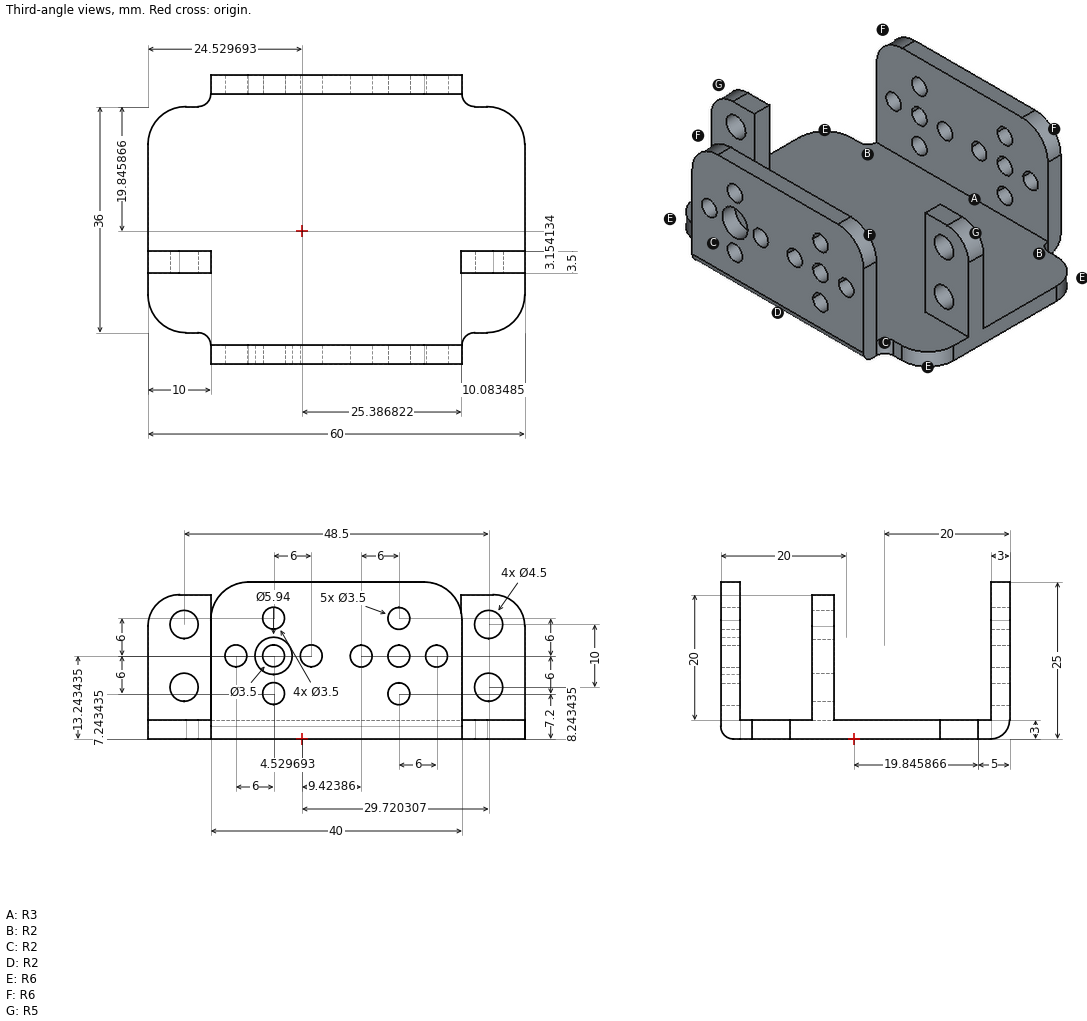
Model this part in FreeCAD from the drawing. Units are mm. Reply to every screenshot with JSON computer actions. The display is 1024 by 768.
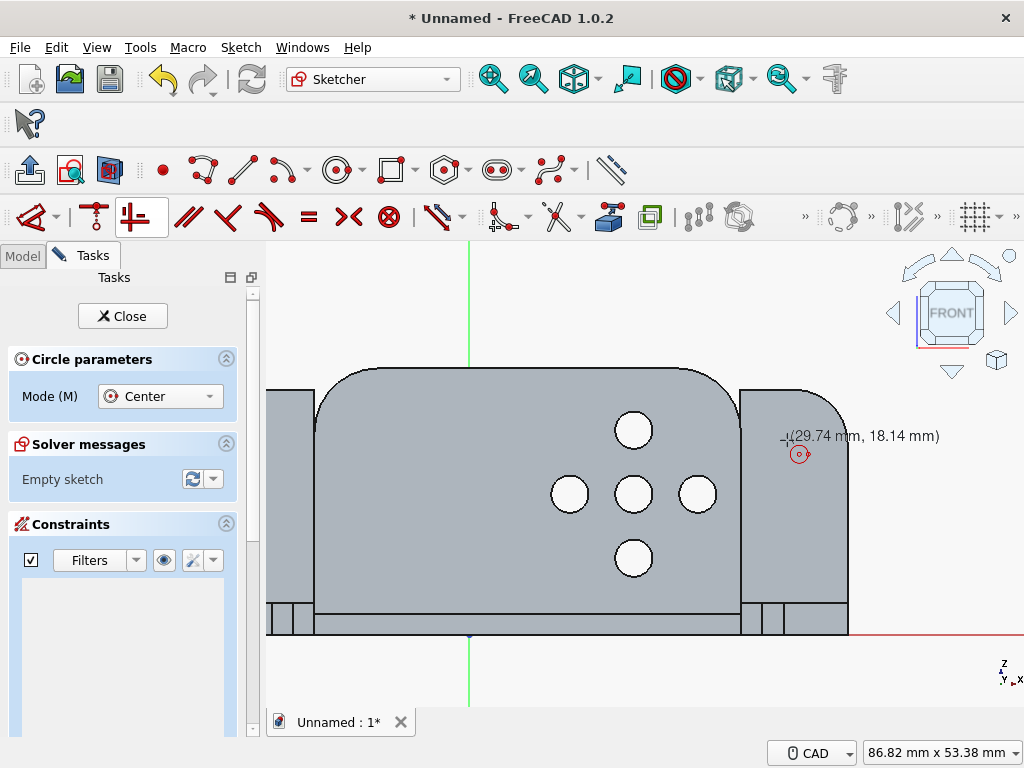
{"action": "left_click", "coordinate": [786, 440]}
{"action": "left_click", "coordinate": [803, 423]}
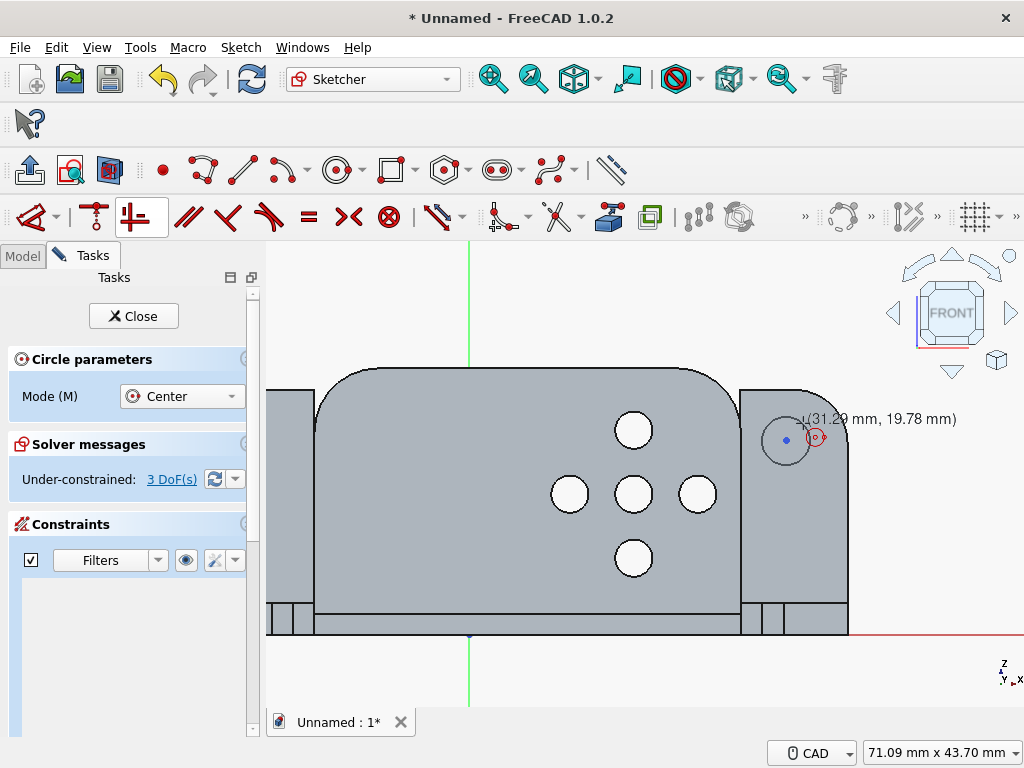
{"action": "left_click", "coordinate": [786, 547]}
{"action": "left_click", "coordinate": [803, 530]}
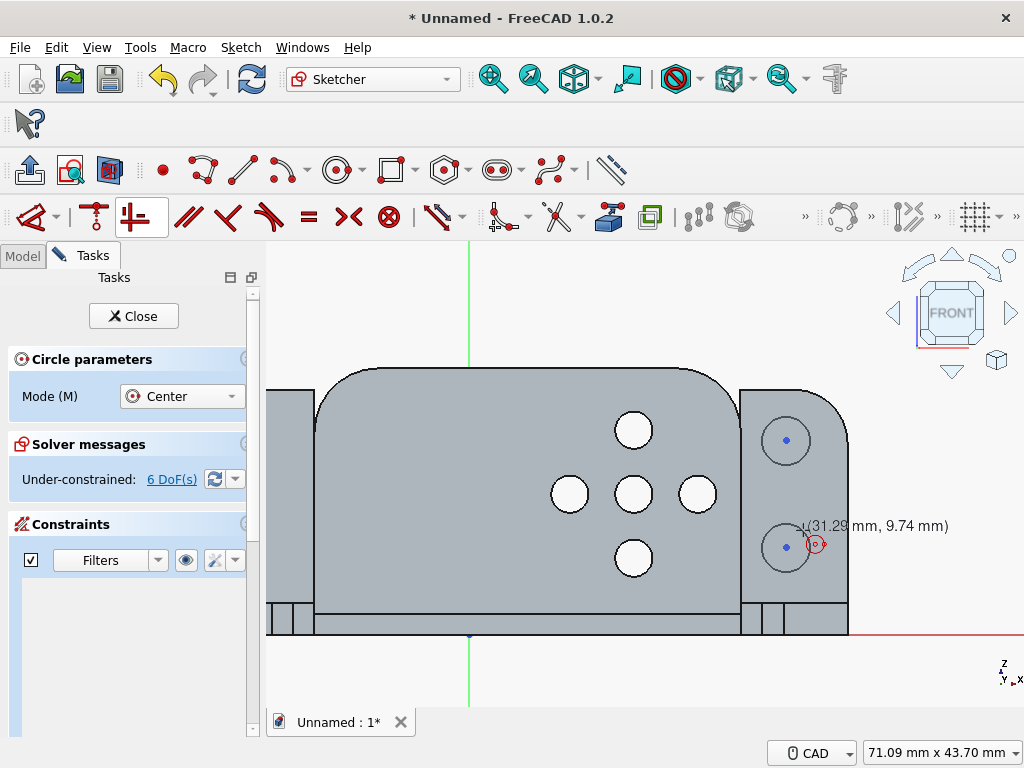
{"action": "scroll", "coordinate": [676, 369], "scroll_direction": "down", "scroll_amount": 2}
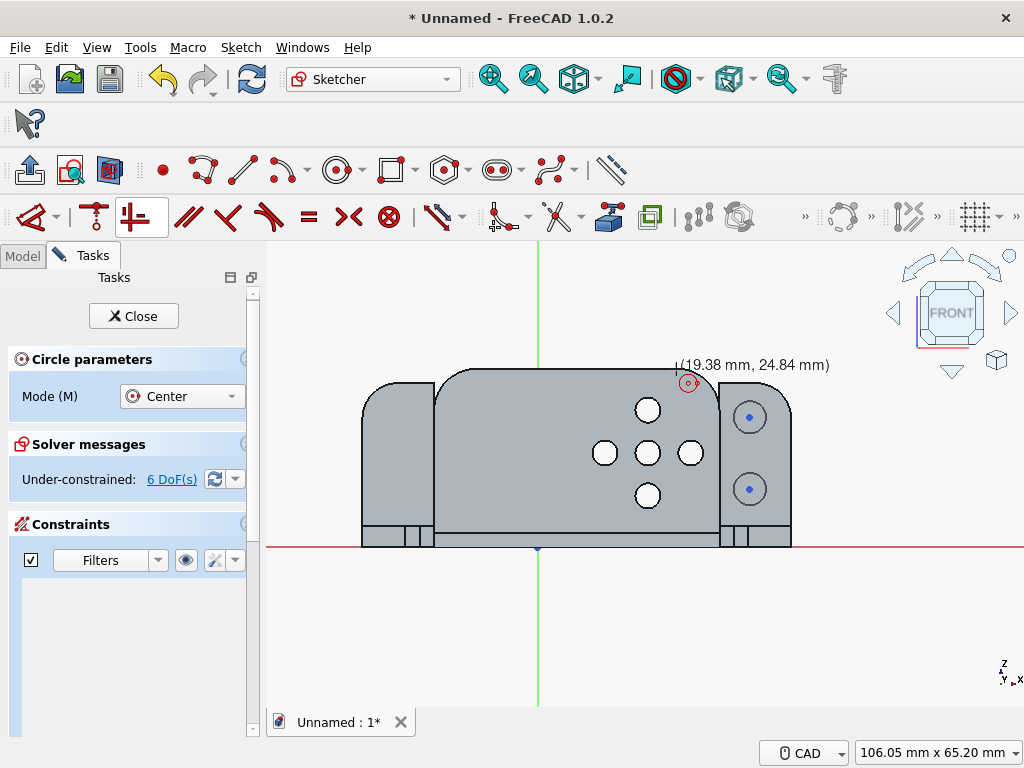
{"action": "scroll", "coordinate": [403, 417], "scroll_direction": "up", "scroll_amount": 2}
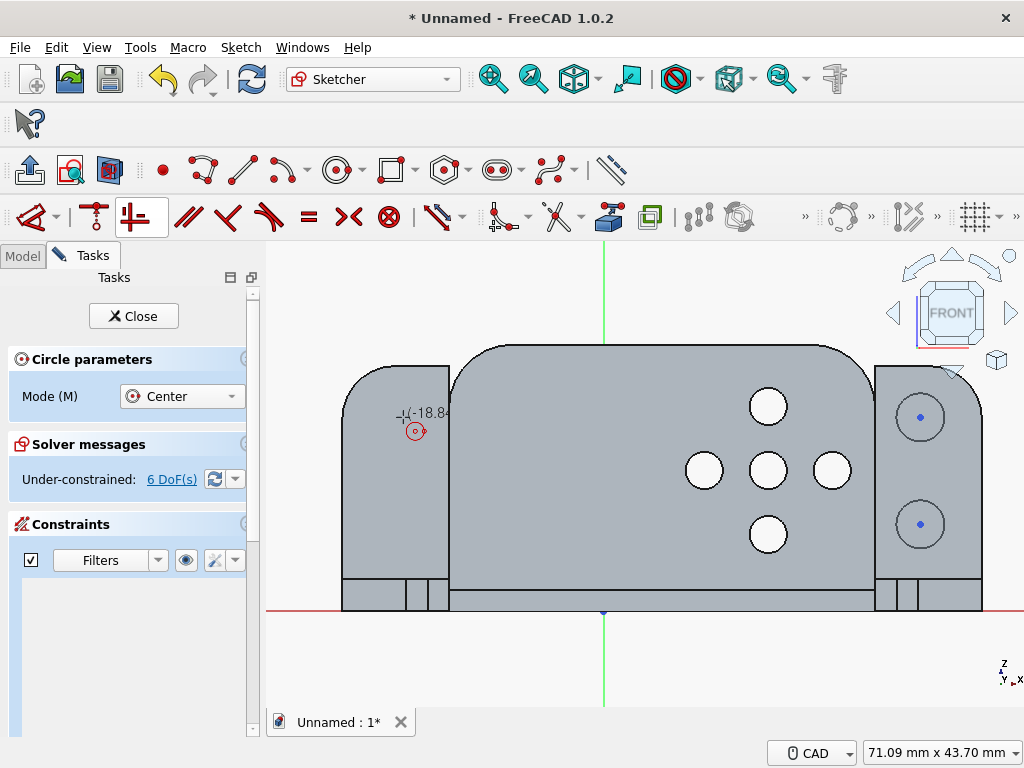
{"action": "left_click", "coordinate": [404, 417]}
{"action": "left_click", "coordinate": [421, 400]}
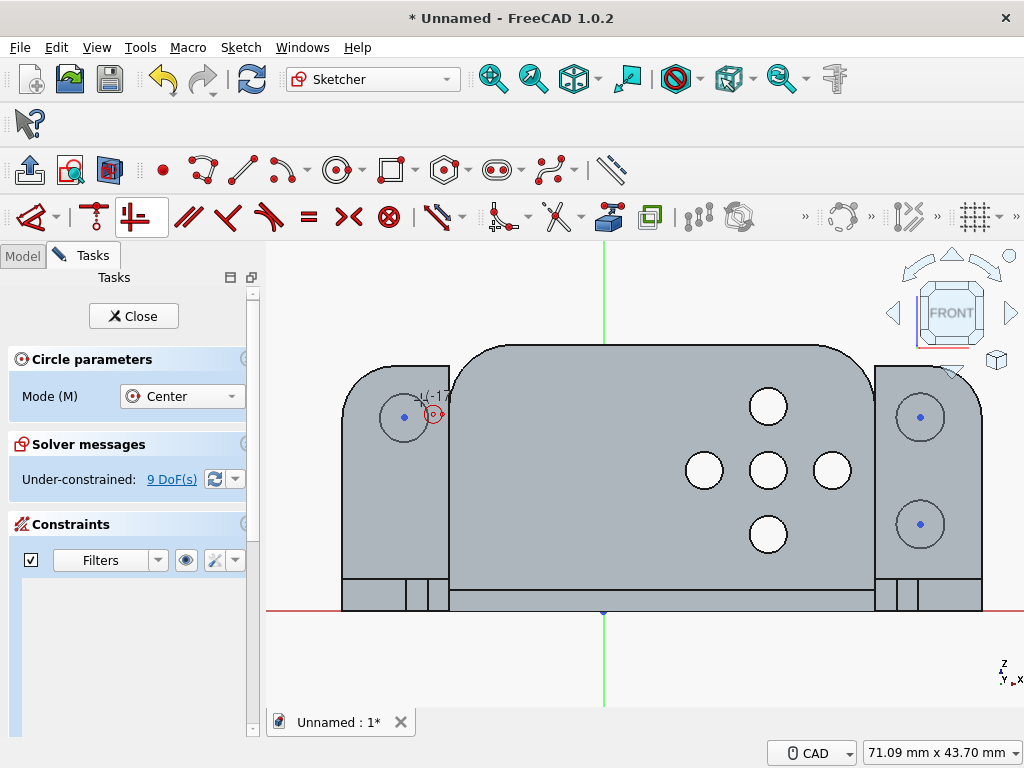
{"action": "left_click", "coordinate": [404, 523]}
{"action": "left_click", "coordinate": [421, 506]}
{"action": "key", "text": "Escape"}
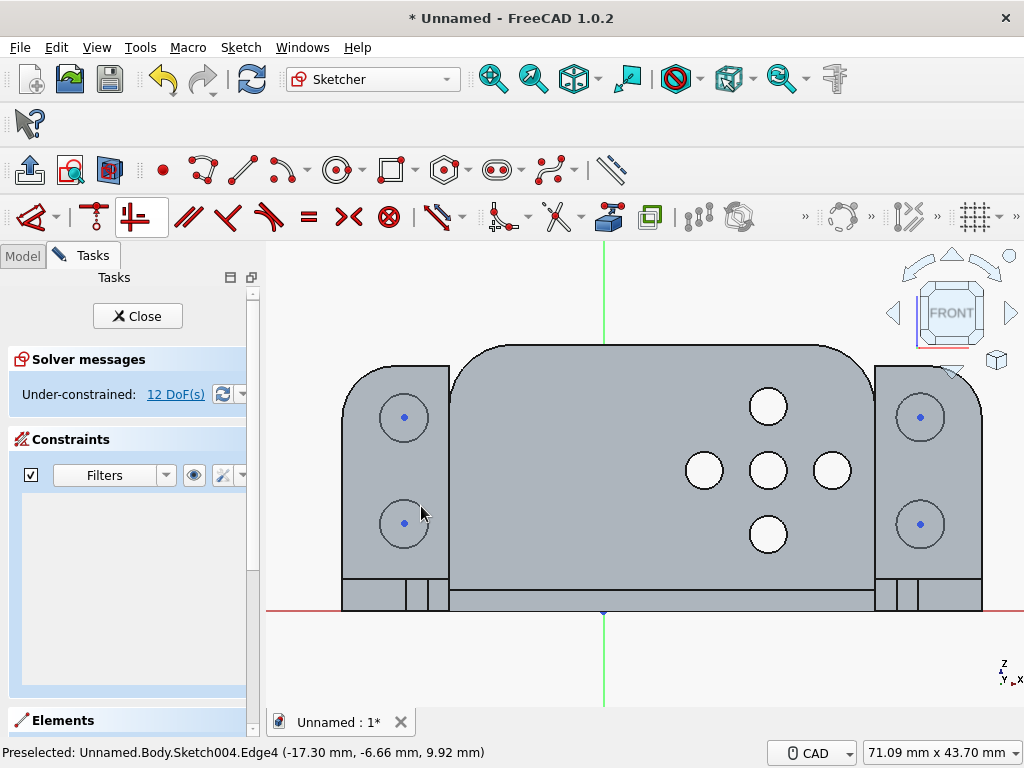
{"action": "scroll", "coordinate": [402, 417], "scroll_direction": "down", "scroll_amount": 2}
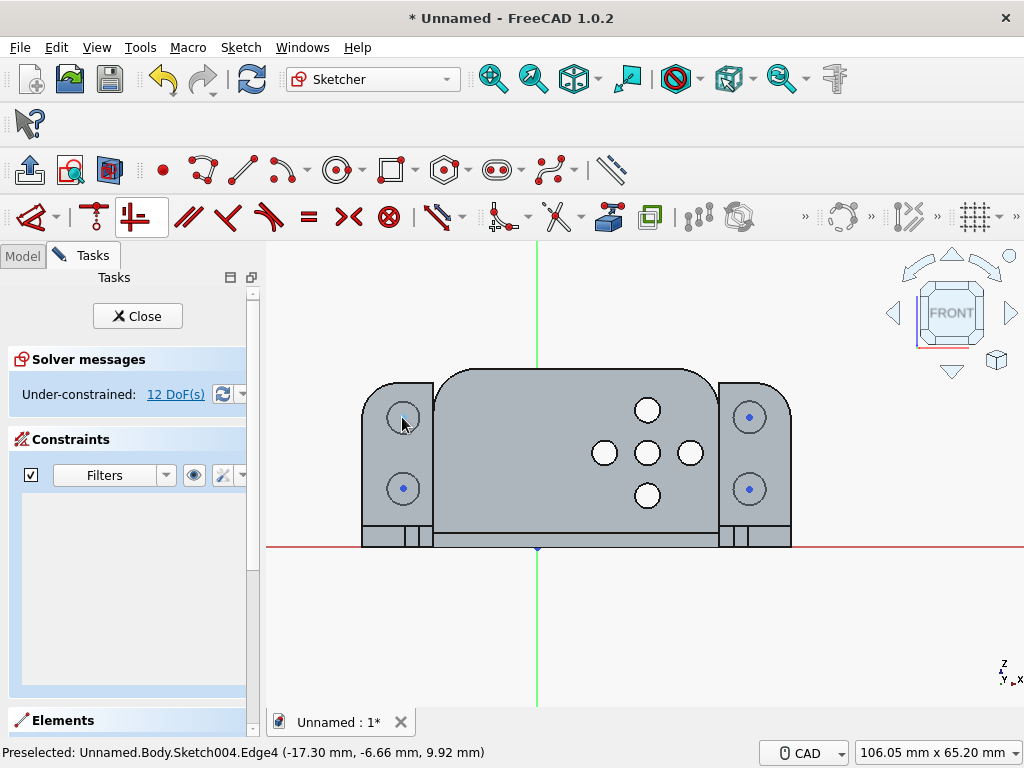
{"action": "left_click", "coordinate": [761, 406]}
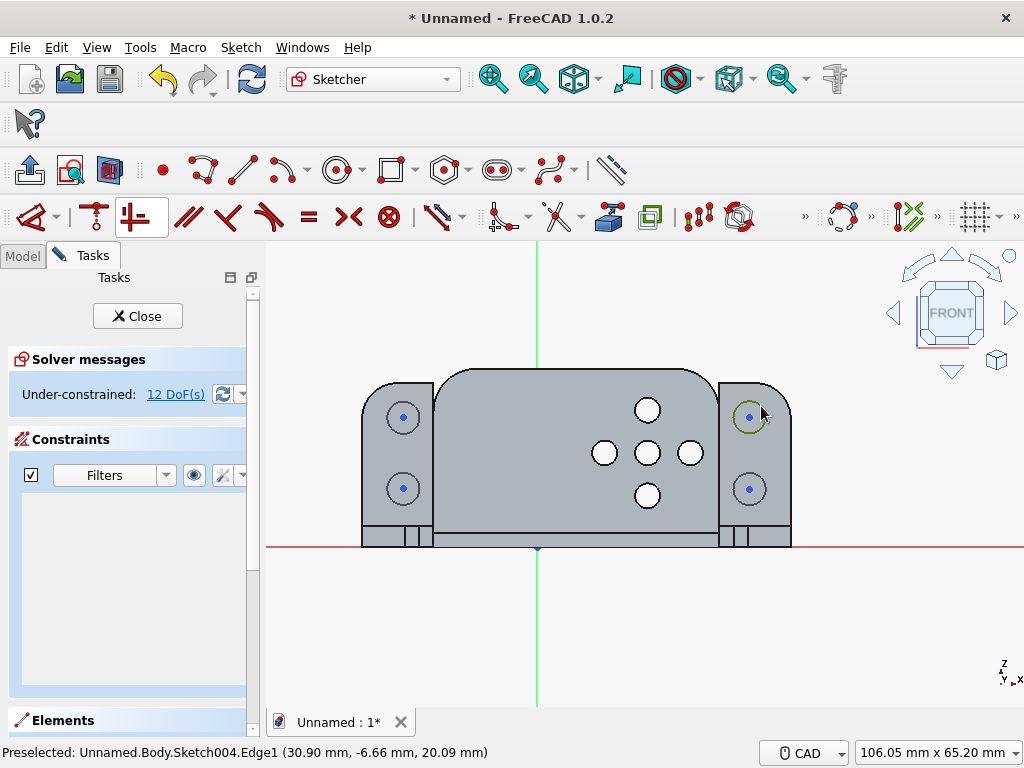
{"action": "left_click", "coordinate": [761, 478]}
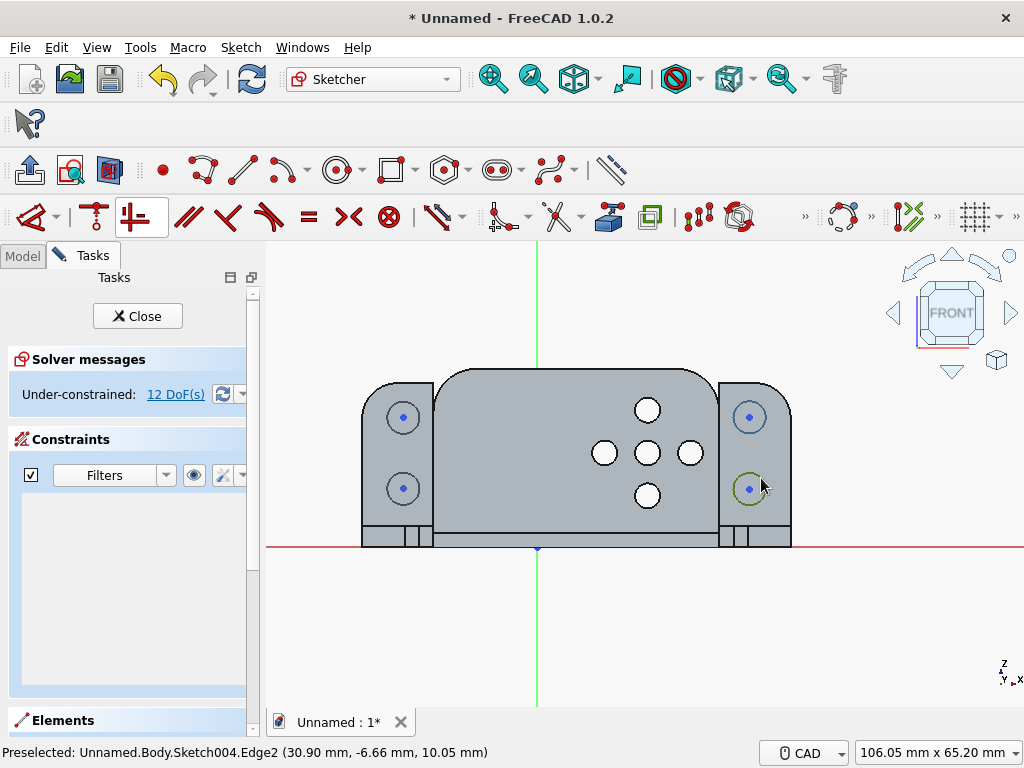
{"action": "left_click", "coordinate": [415, 406]}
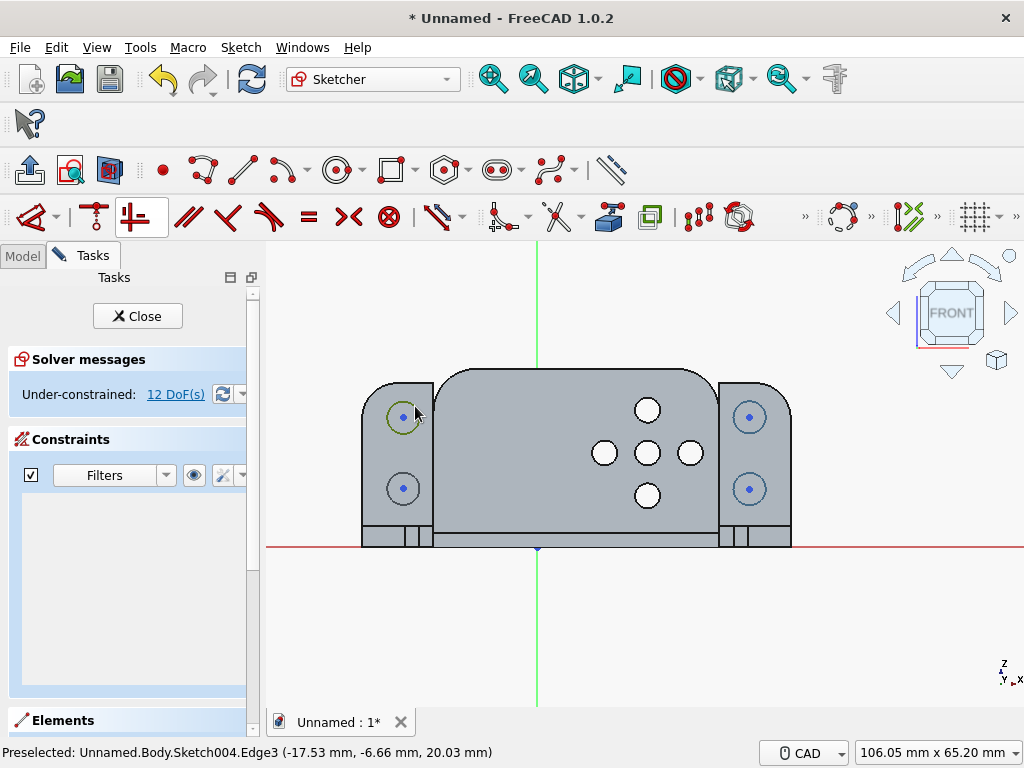
{"action": "left_click", "coordinate": [415, 477]}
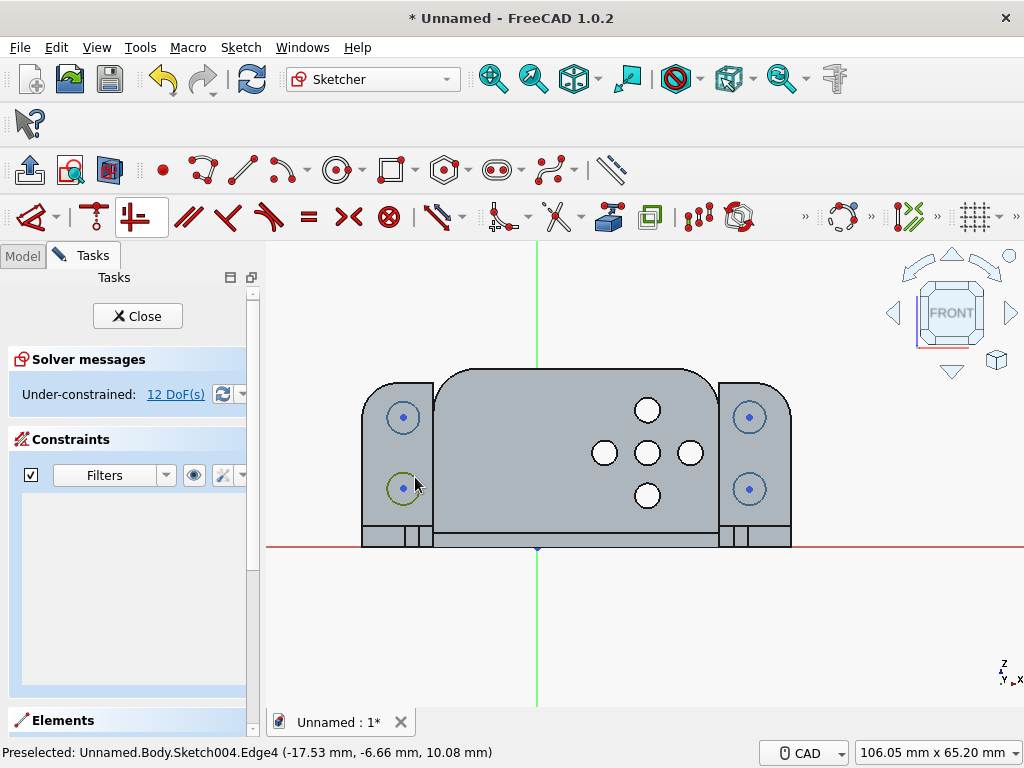
{"action": "left_click", "coordinate": [310, 218]}